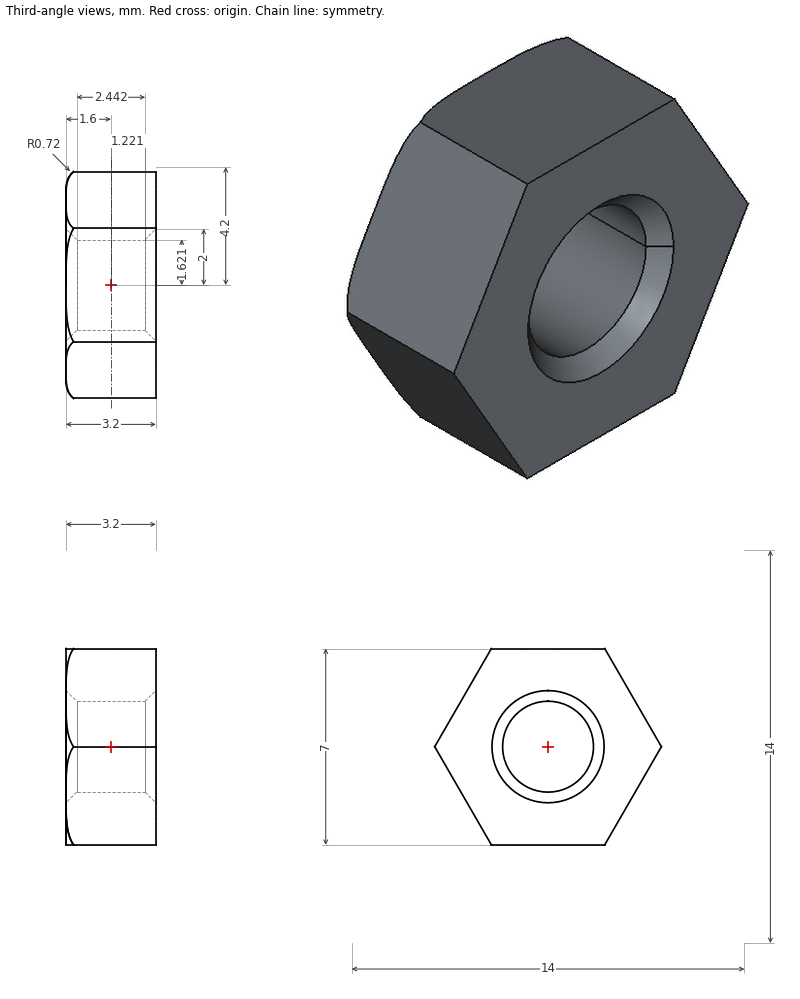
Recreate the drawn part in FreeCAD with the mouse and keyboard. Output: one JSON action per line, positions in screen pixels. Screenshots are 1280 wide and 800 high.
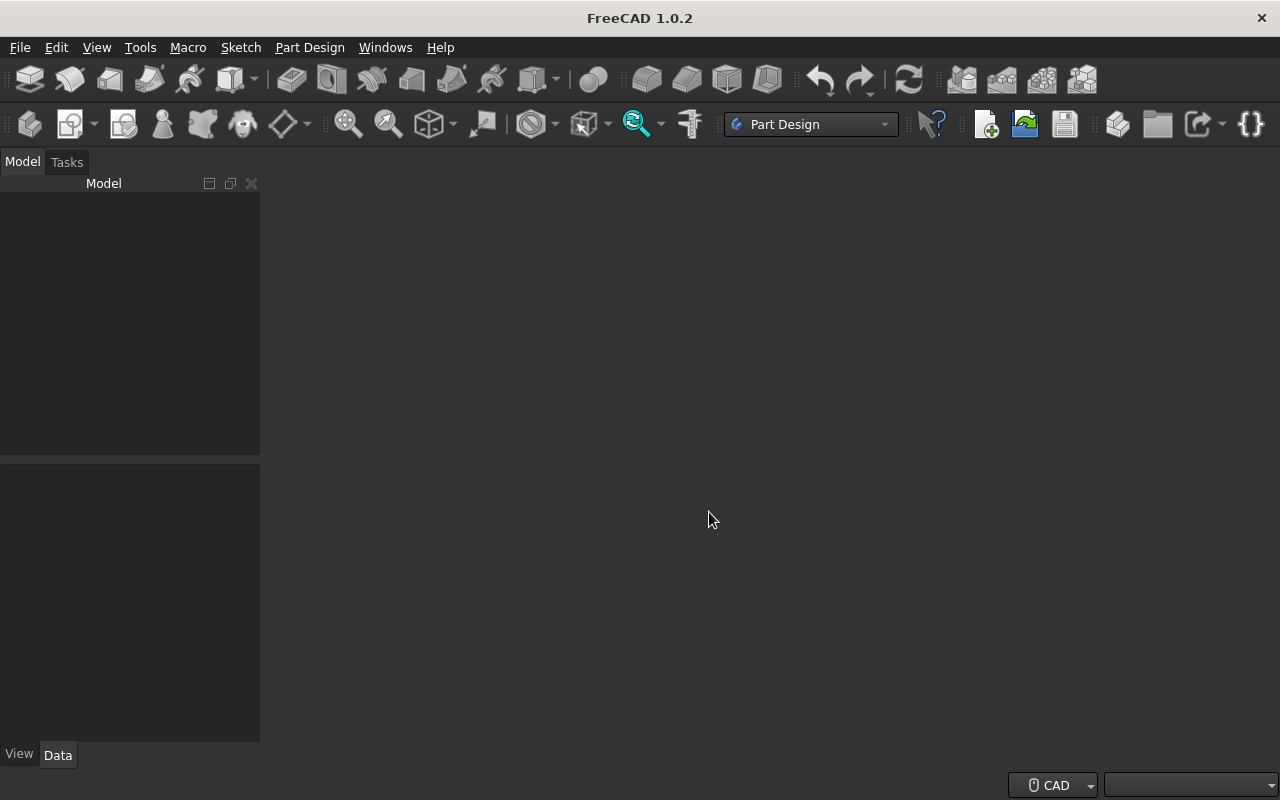
{"action": "key", "text": "ctrl+n"}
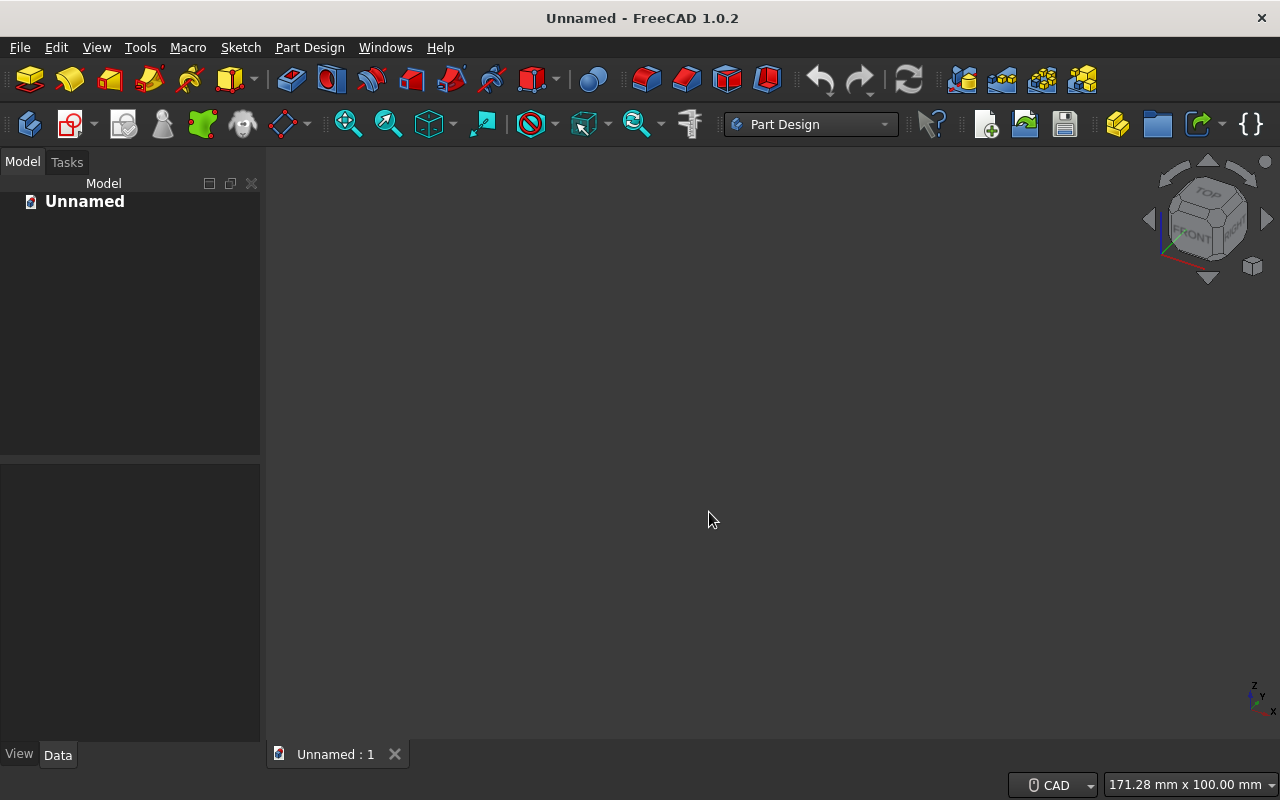
{"action": "left_click", "coordinate": [70, 124]}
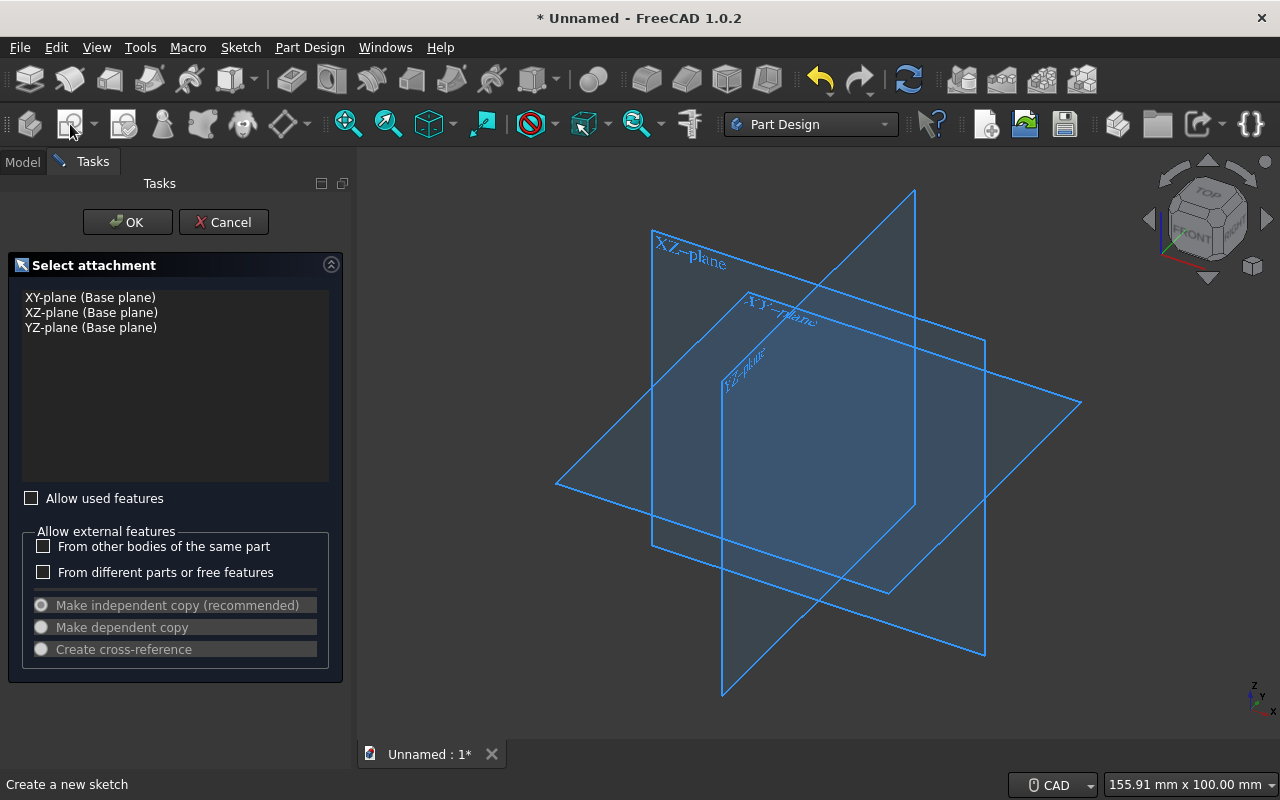
{"action": "left_click", "coordinate": [82, 298]}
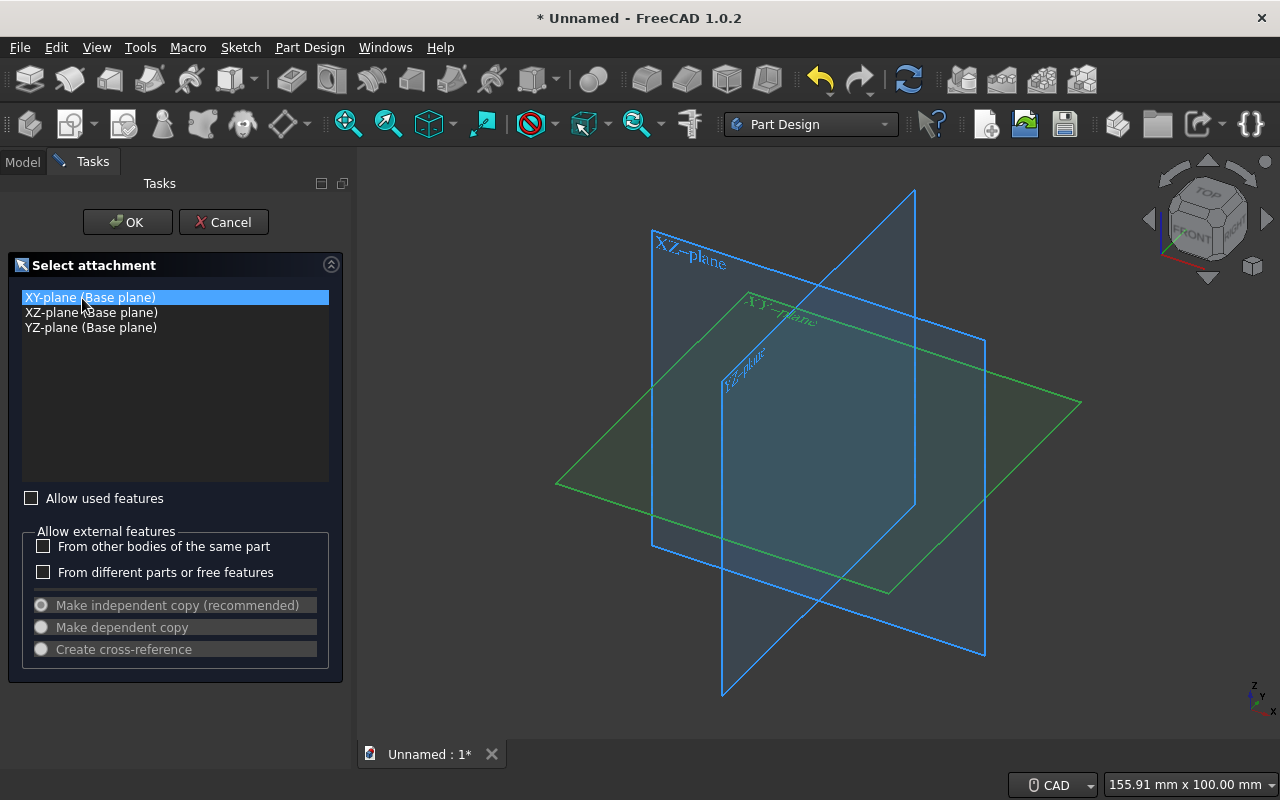
{"action": "left_click", "coordinate": [128, 222]}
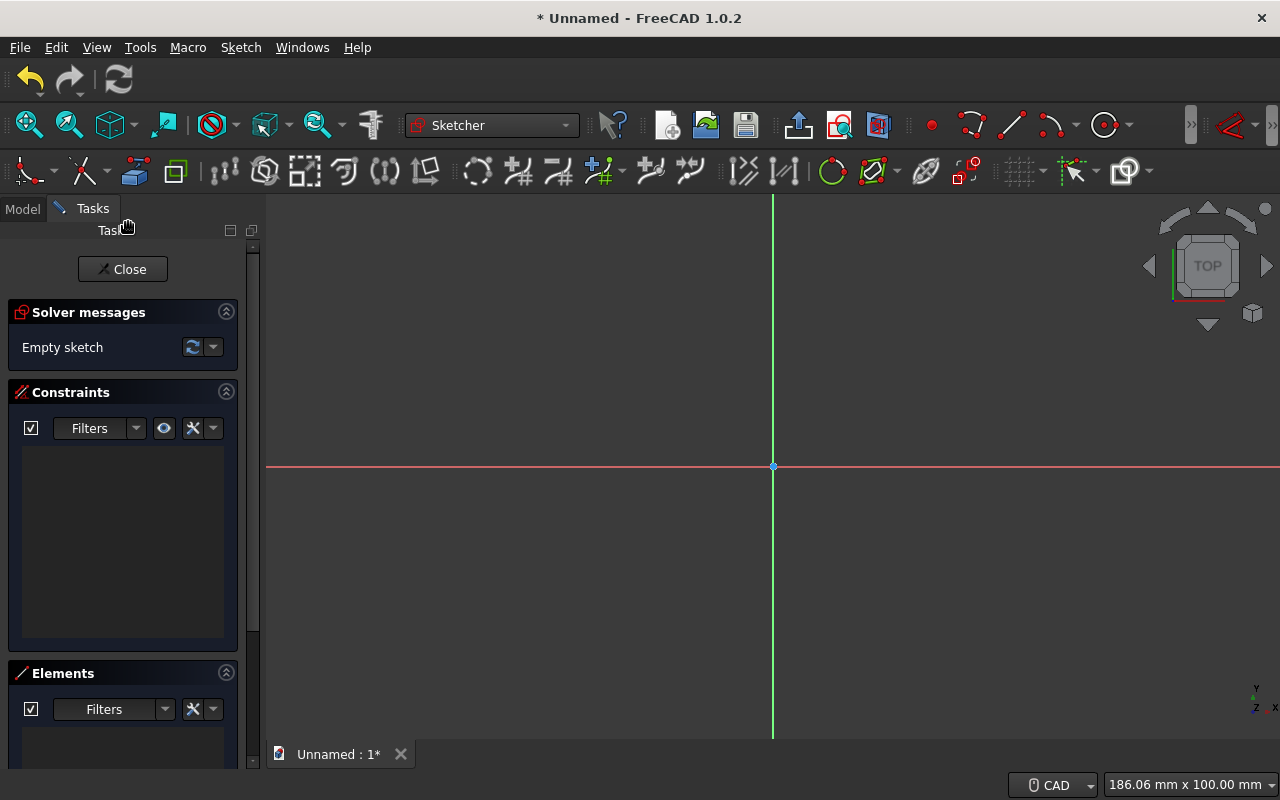
{"action": "scroll", "coordinate": [777, 454], "scroll_direction": "up", "scroll_amount": 14}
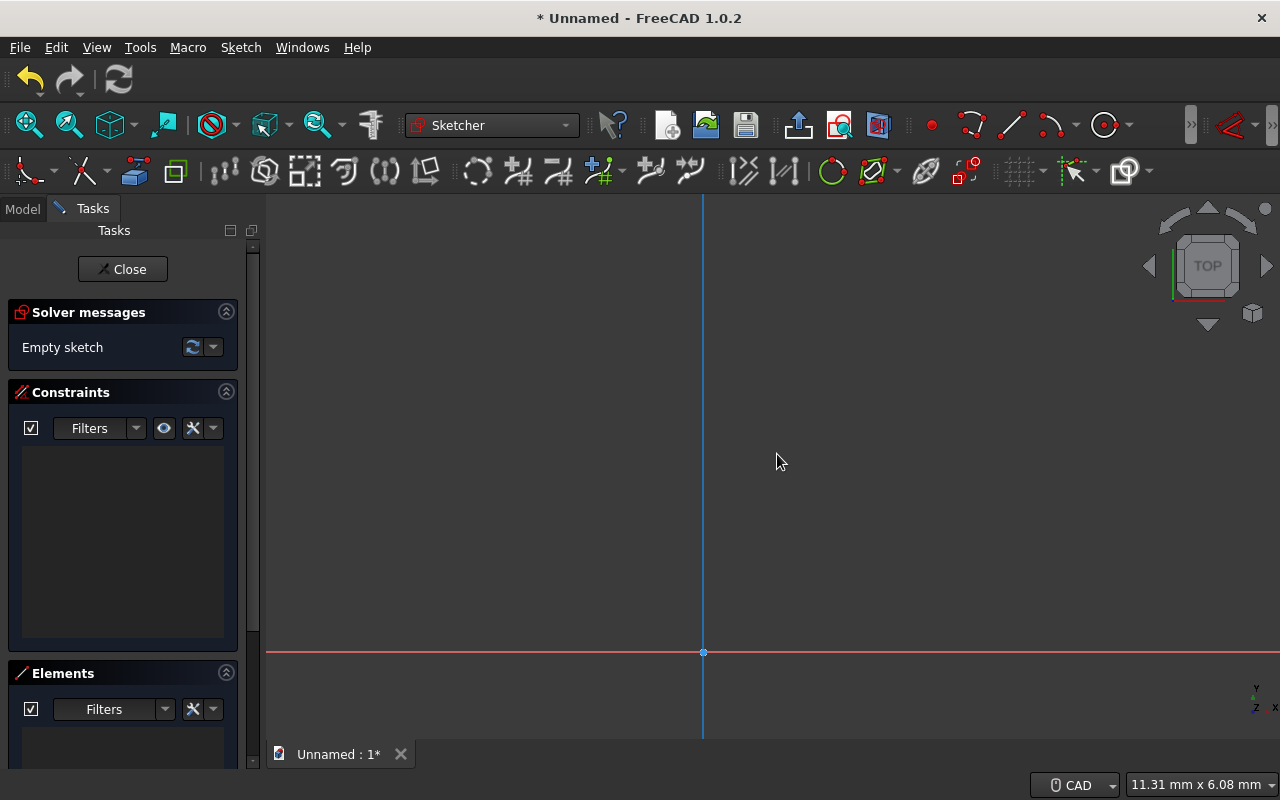
{"action": "left_click", "coordinate": [972, 126]}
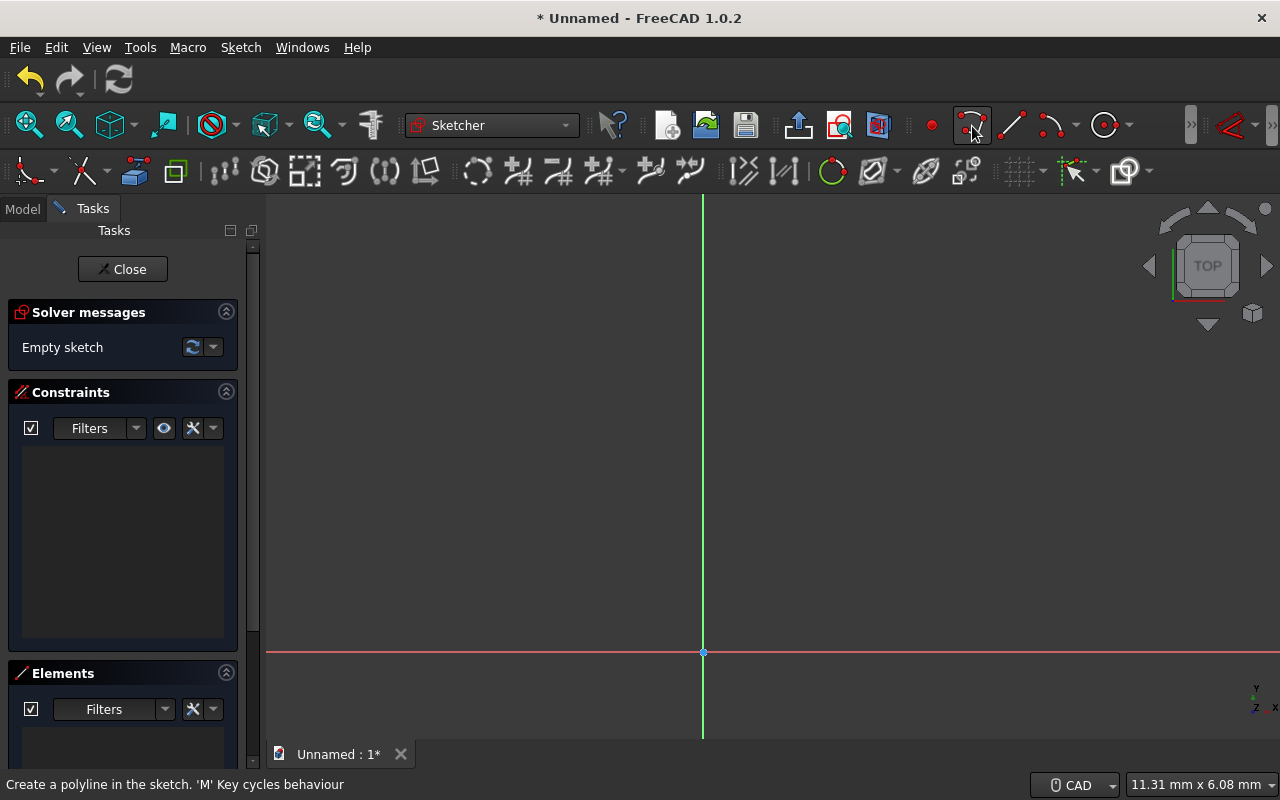
{"action": "left_click", "coordinate": [560, 340]}
{"action": "left_click", "coordinate": [560, 652]}
{"action": "left_click", "coordinate": [847, 643]}
{"action": "left_click", "coordinate": [847, 276]}
{"action": "left_click", "coordinate": [625, 276]}
{"action": "right_click", "coordinate": [625, 276]}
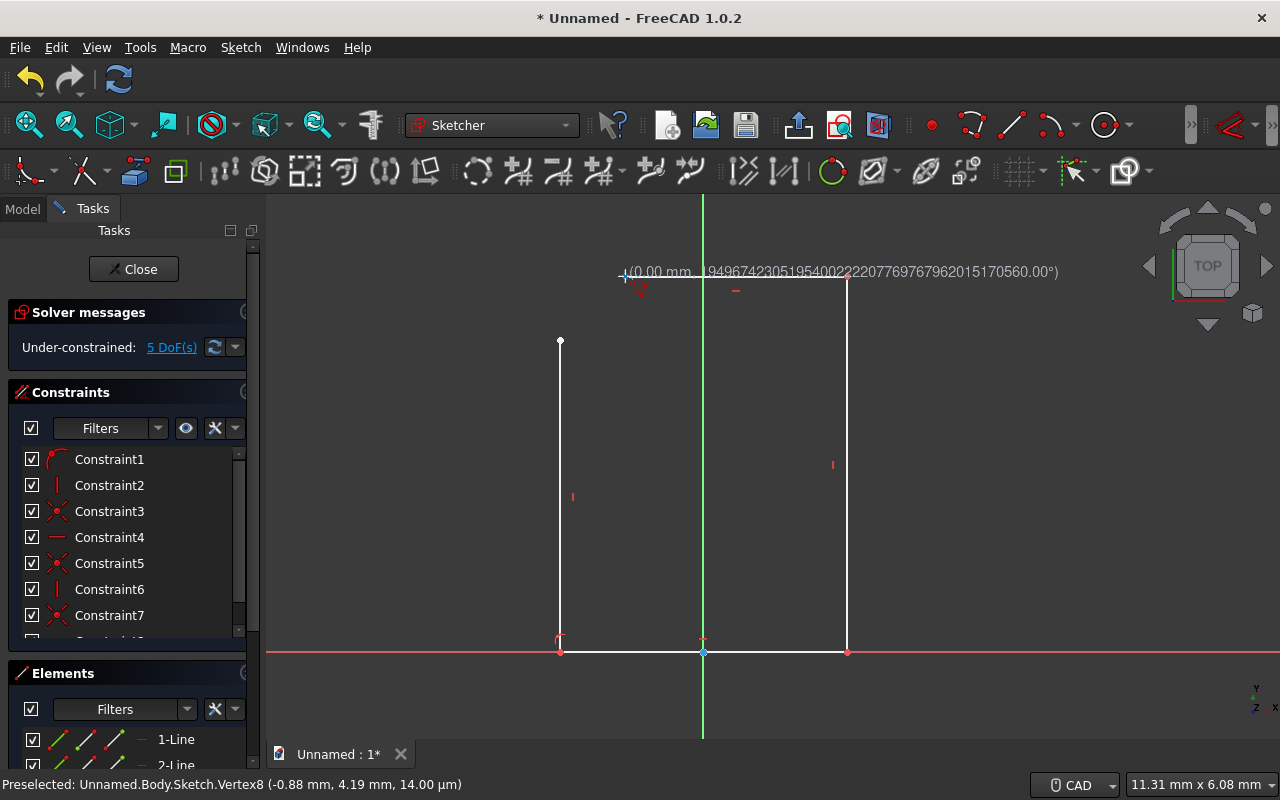
{"action": "key", "text": "g 3 a"}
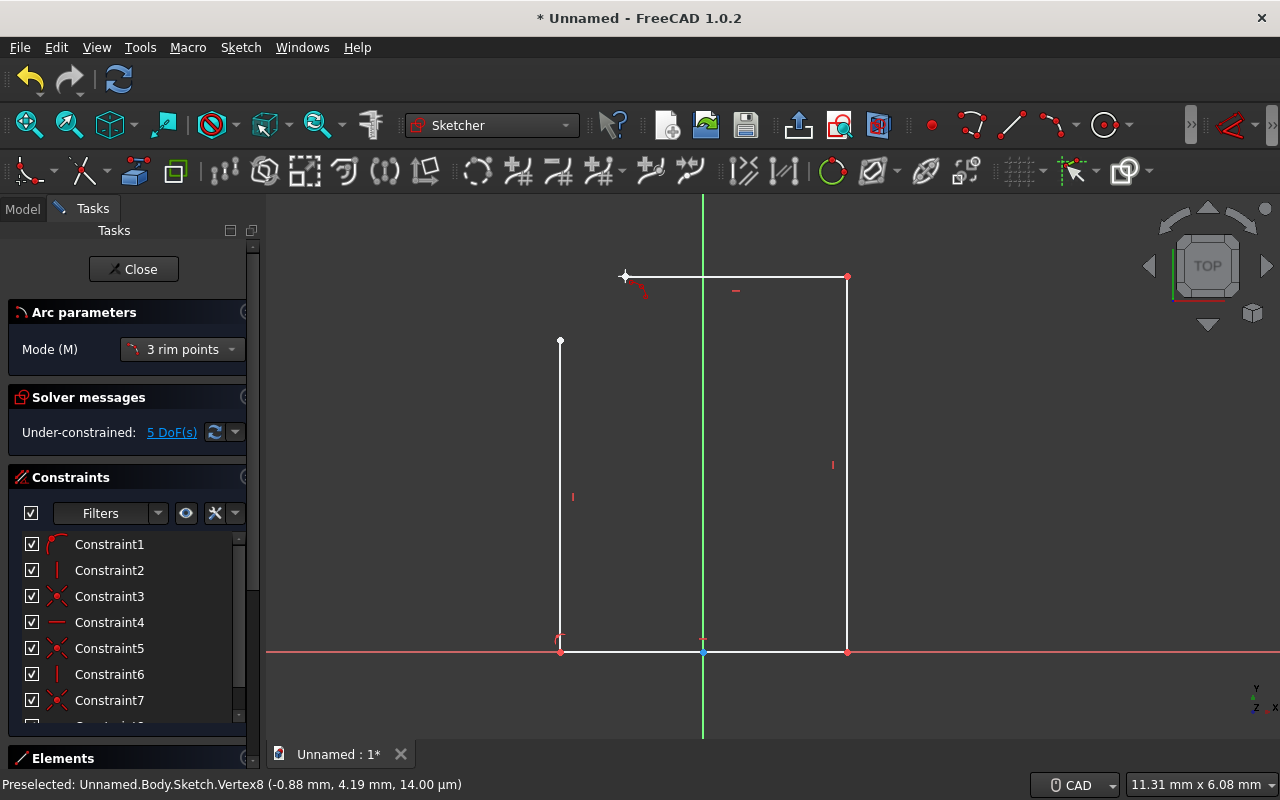
{"action": "left_click", "coordinate": [625, 277]}
{"action": "left_click", "coordinate": [560, 341]}
{"action": "left_click", "coordinate": [579, 295]}
{"action": "key", "text": "Escape"}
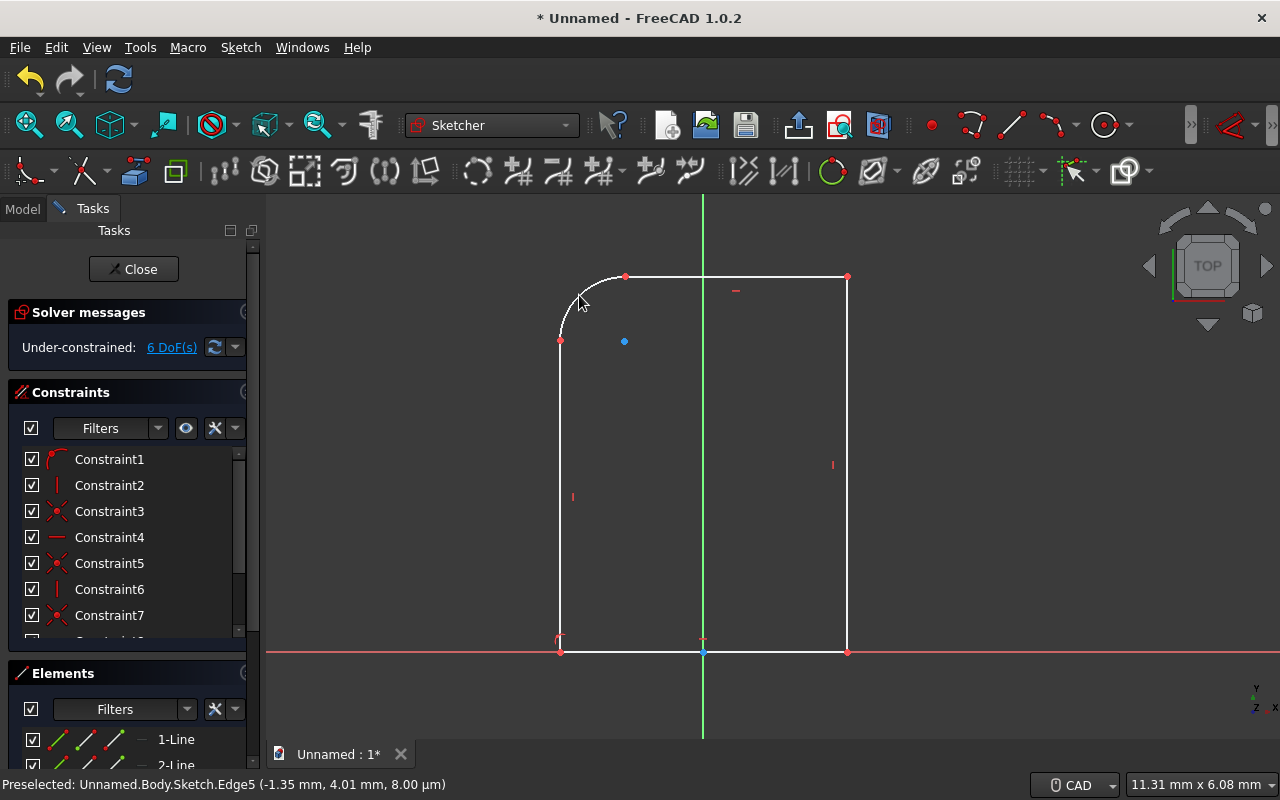
{"action": "left_click", "coordinate": [560, 434]}